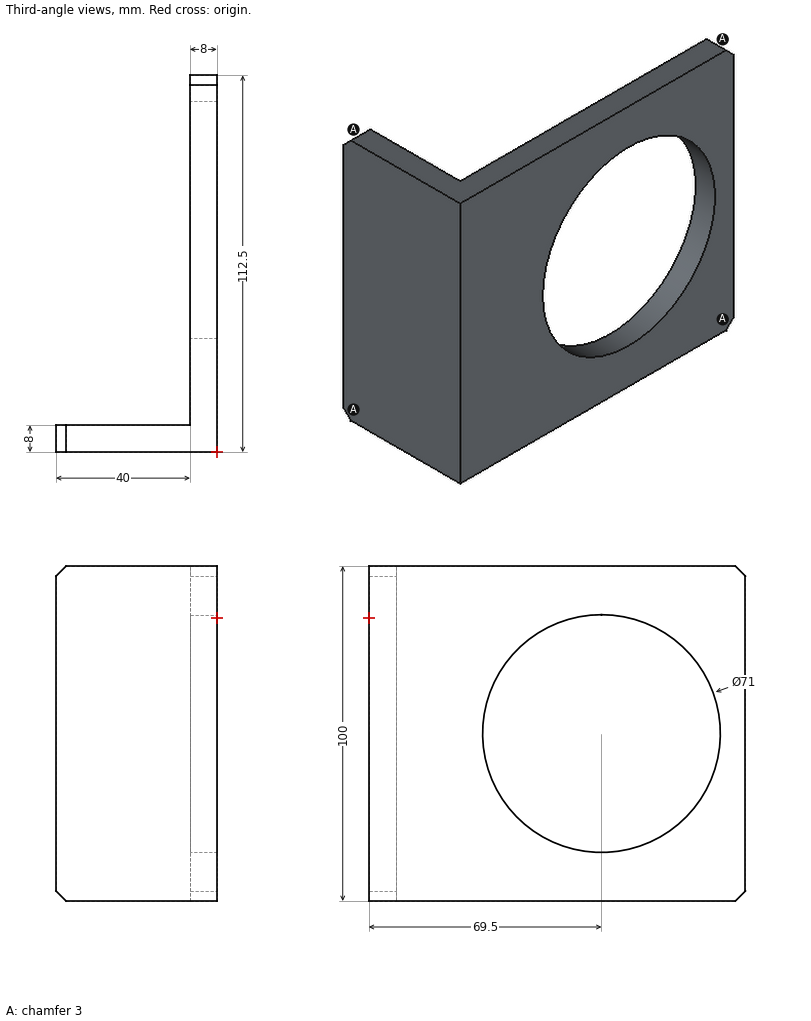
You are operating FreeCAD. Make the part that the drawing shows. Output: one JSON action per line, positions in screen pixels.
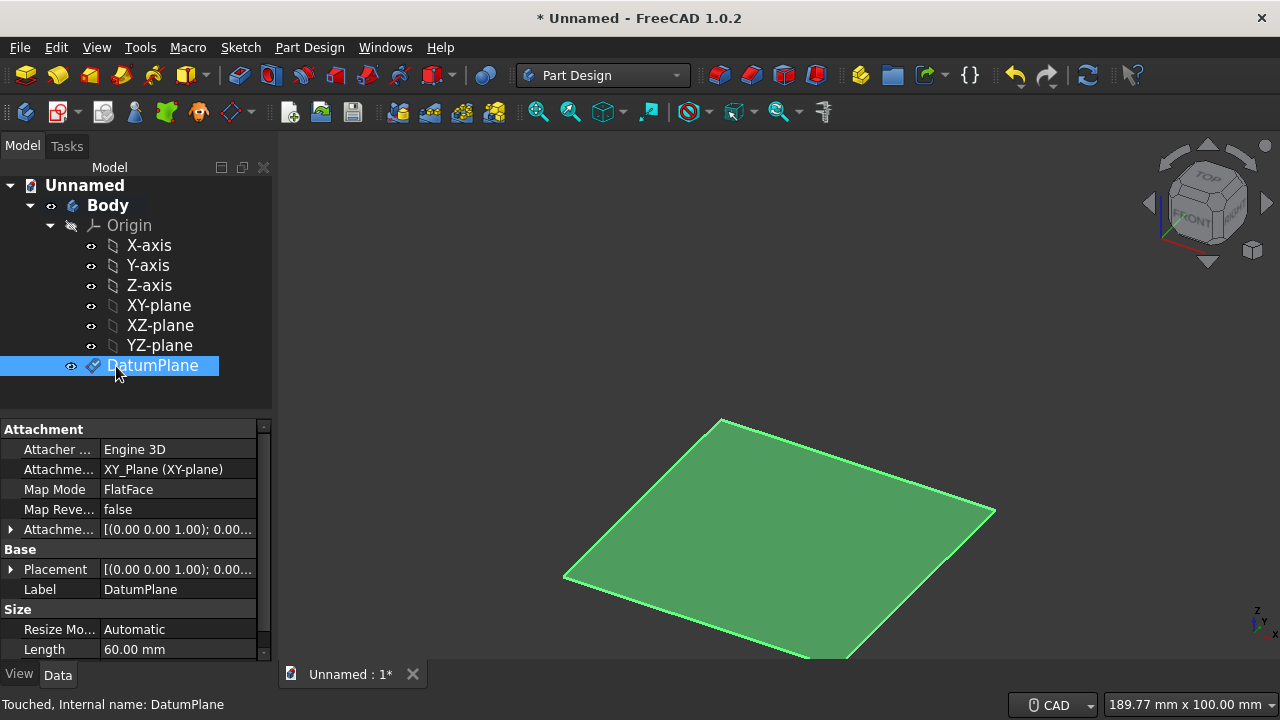
{"action": "left_click", "coordinate": [58, 112]}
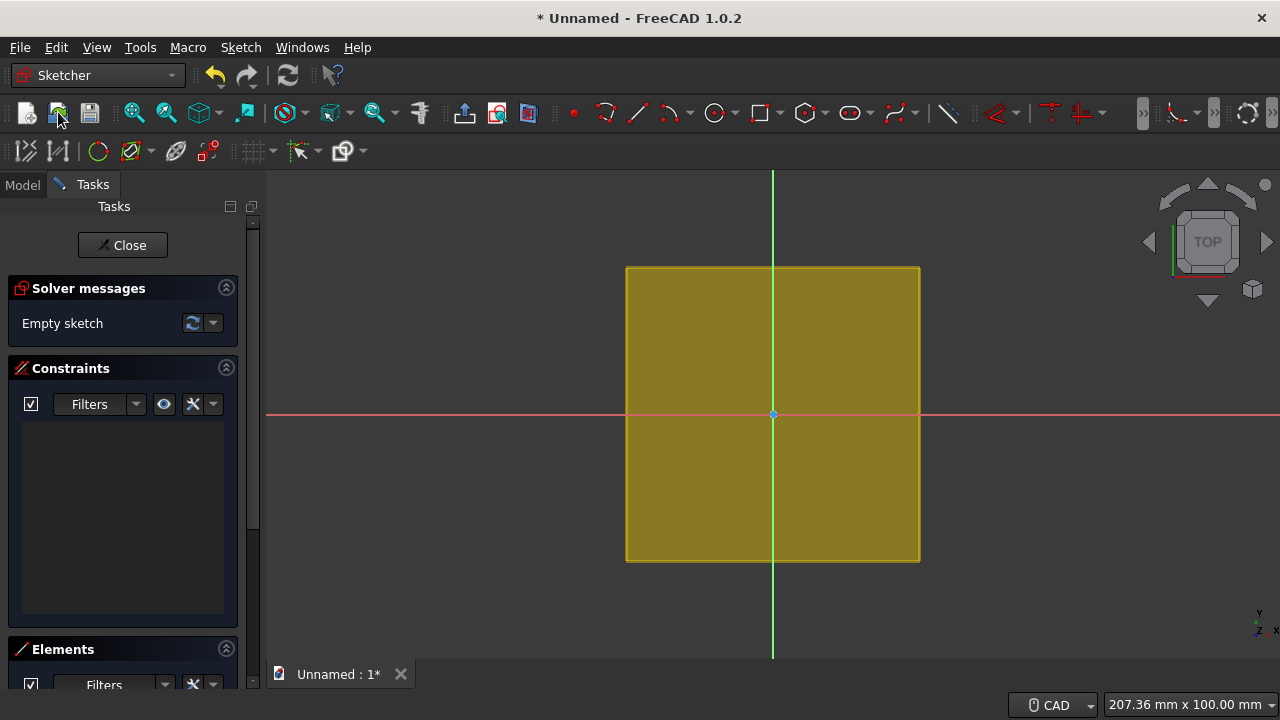
{"action": "scroll", "coordinate": [744, 631], "scroll_direction": "down", "scroll_amount": 4}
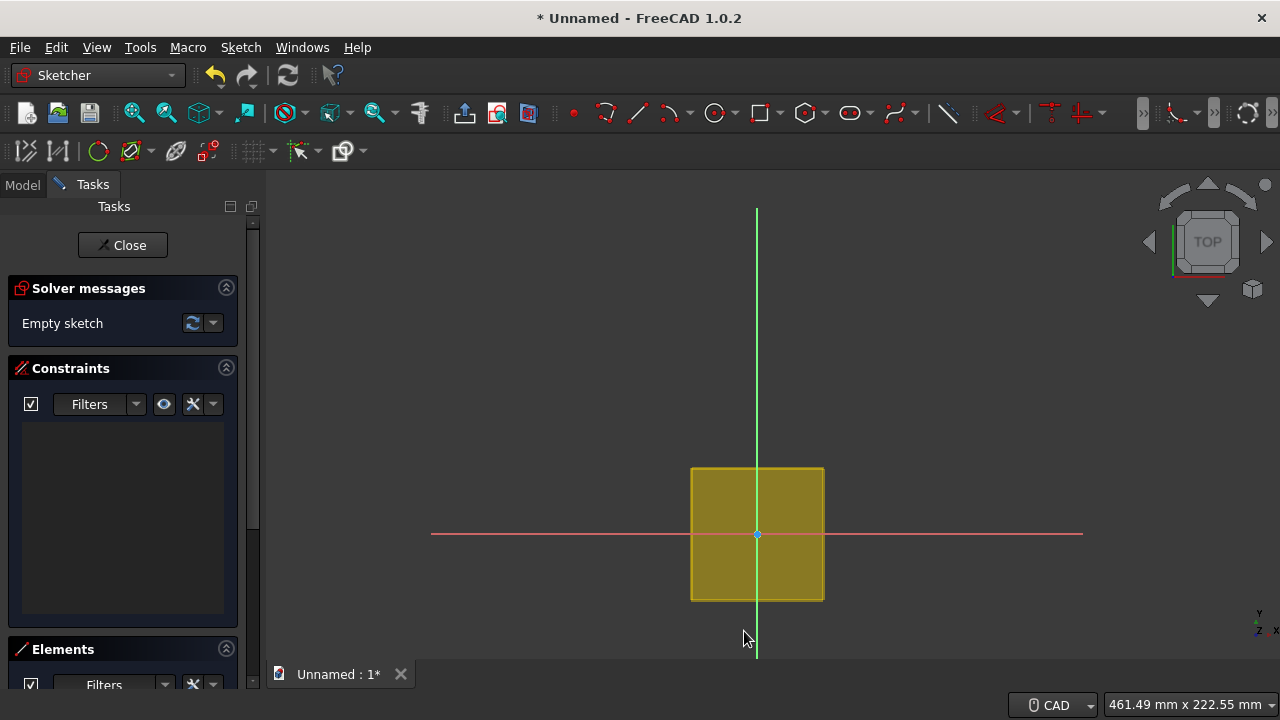
{"action": "left_click", "coordinate": [606, 114]}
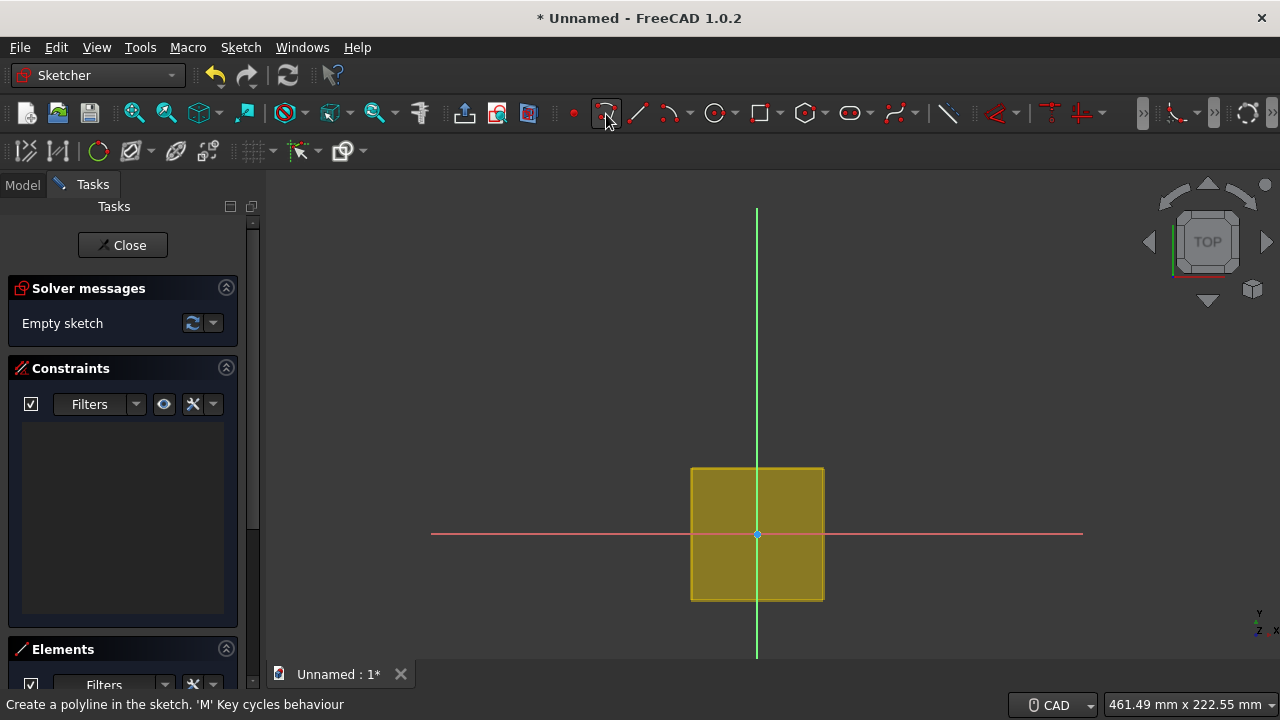
{"action": "left_click", "coordinate": [757, 534]}
{"action": "left_click", "coordinate": [748, 287]}
{"action": "left_click", "coordinate": [740, 287]}
{"action": "left_click", "coordinate": [740, 517]}
{"action": "left_click", "coordinate": [652, 517]}
{"action": "left_click", "coordinate": [652, 525]}
{"action": "left_click", "coordinate": [757, 534]}
{"action": "key", "text": "Escape"}
{"action": "key", "text": "Escape"}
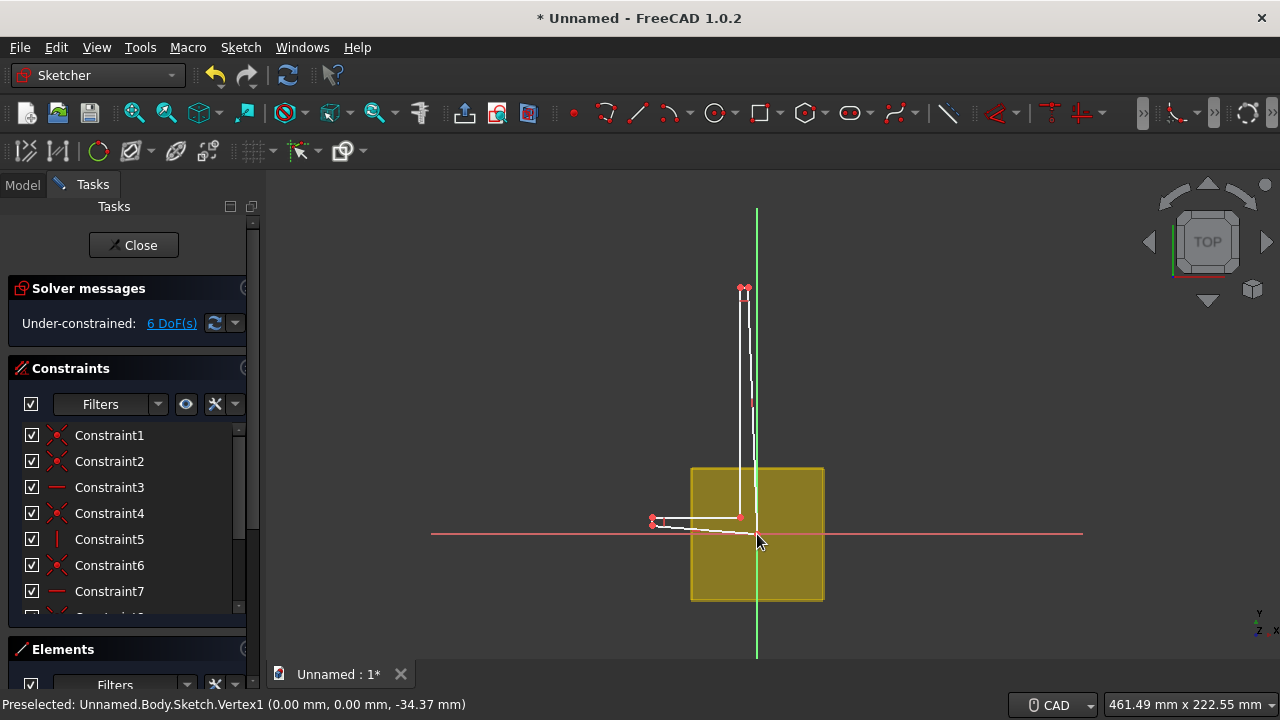
{"action": "left_click", "coordinate": [755, 460]}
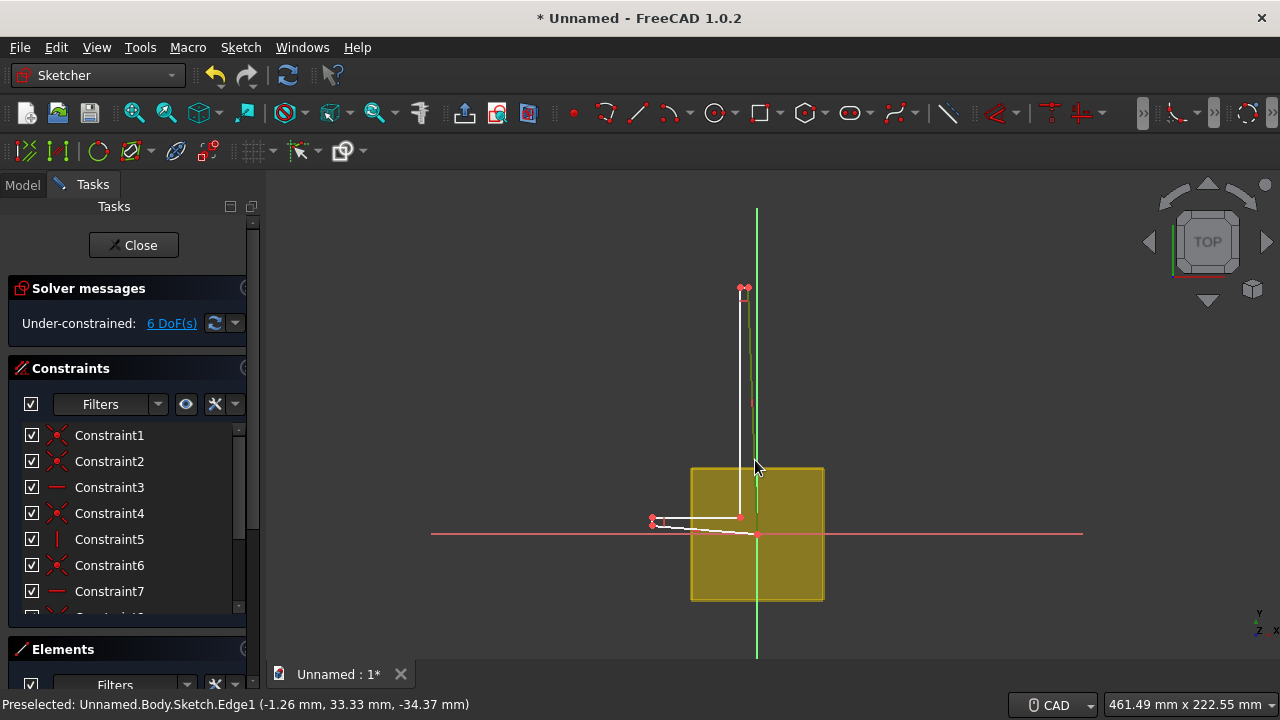
{"action": "key", "text": "v"}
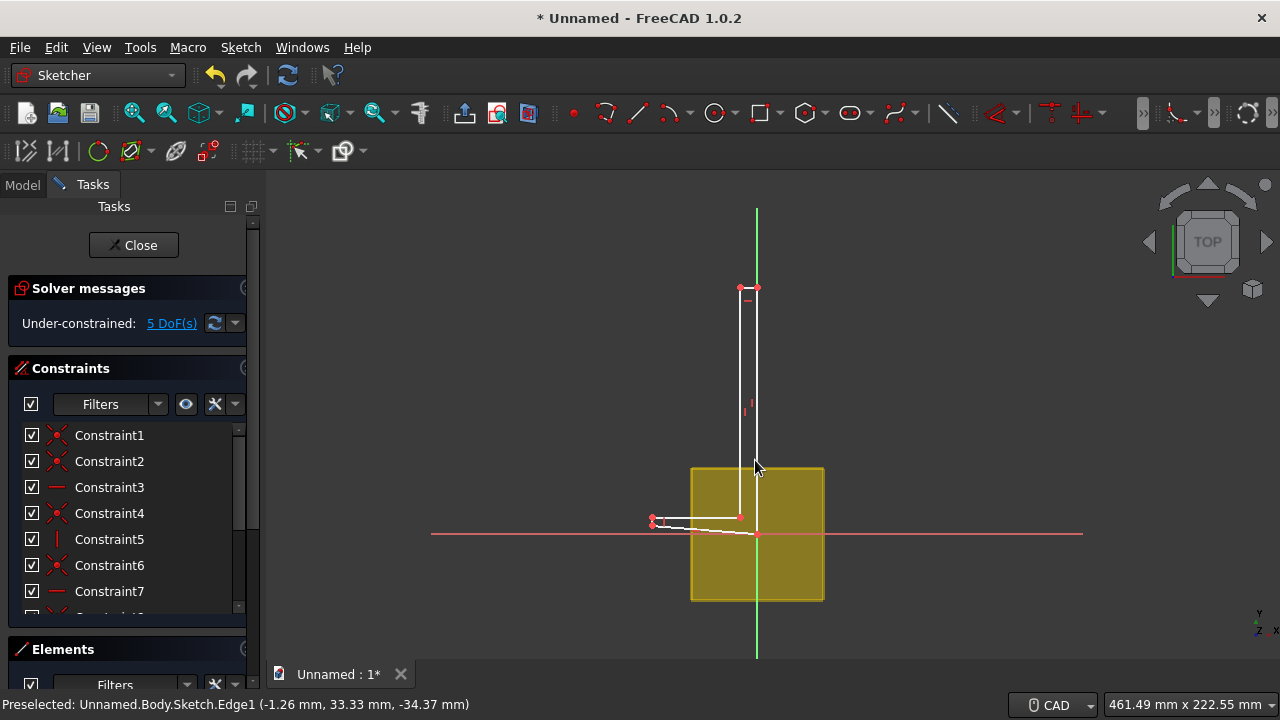
{"action": "left_click", "coordinate": [726, 532]}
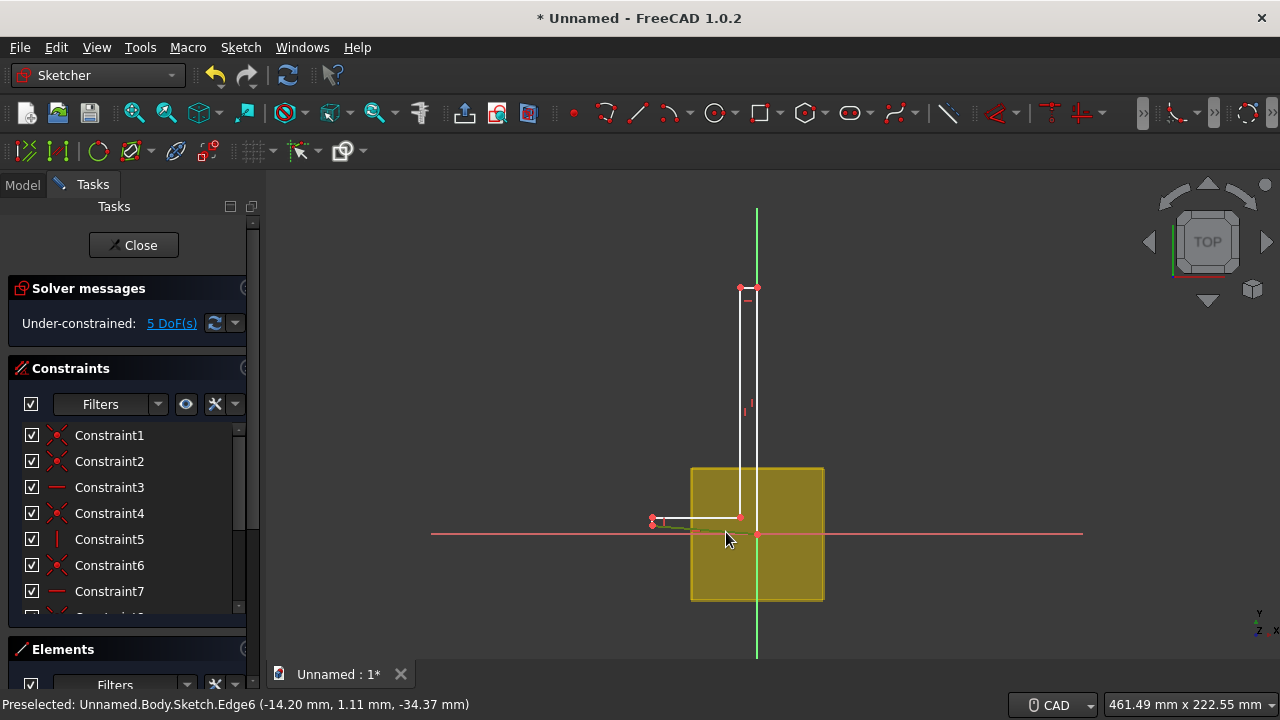
{"action": "left_click", "coordinate": [1104, 114]}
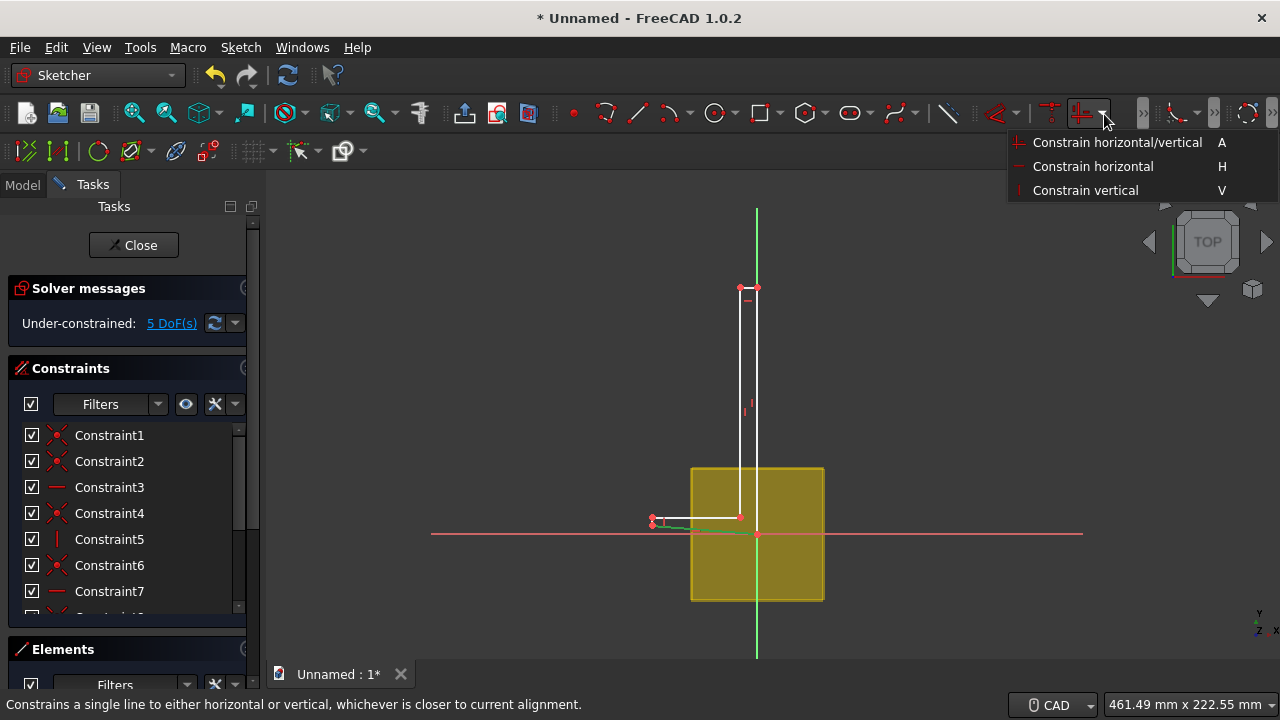
{"action": "left_click", "coordinate": [1143, 166]}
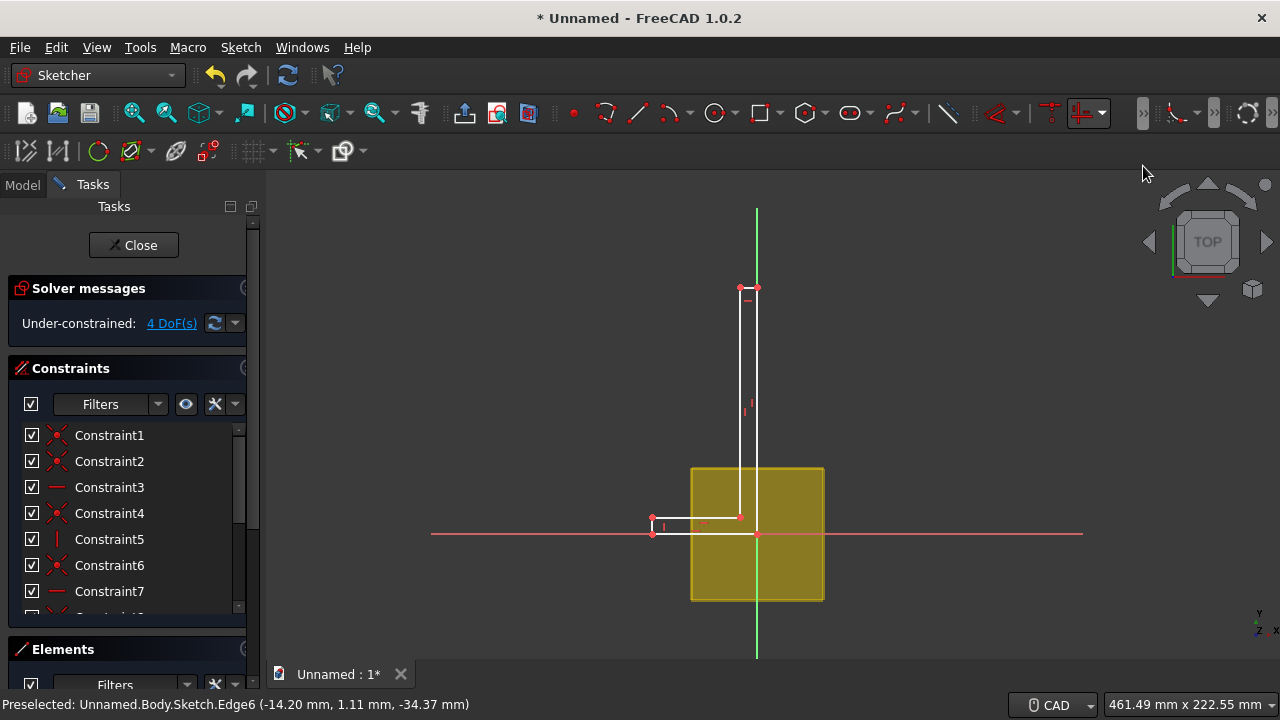
{"action": "scroll", "coordinate": [749, 288], "scroll_direction": "up", "scroll_amount": 5}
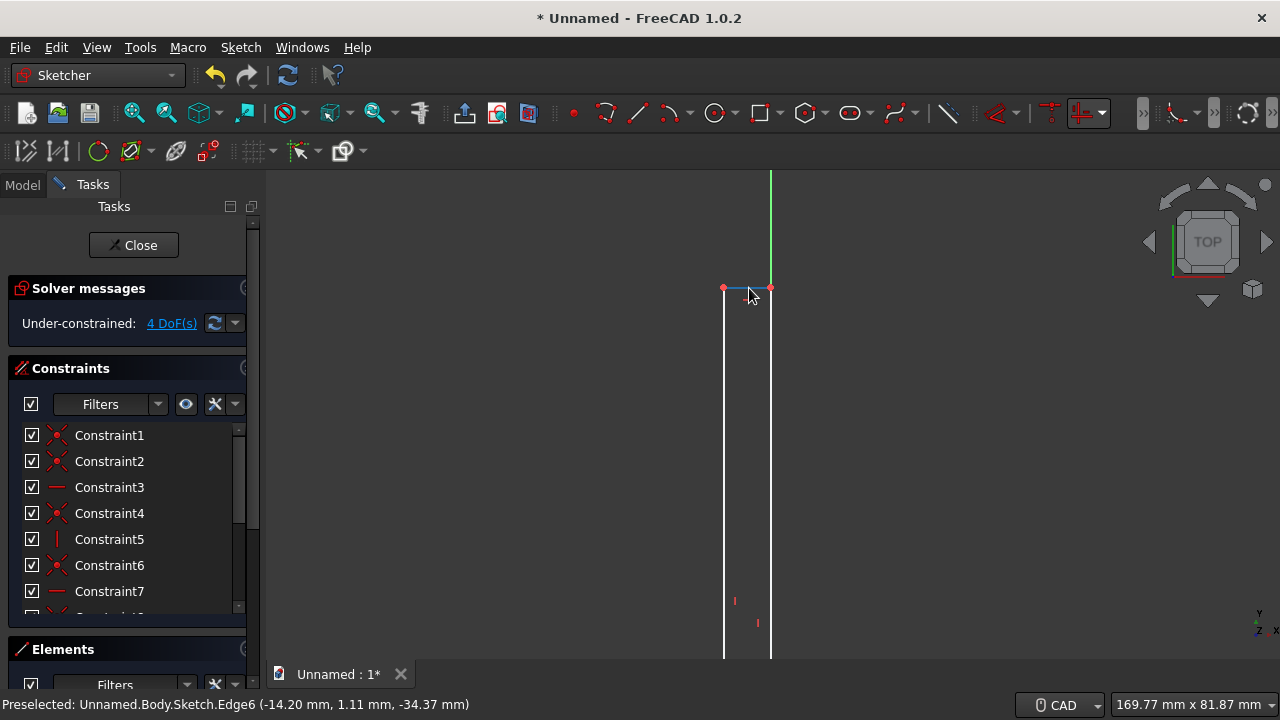
{"action": "left_click", "coordinate": [747, 288]}